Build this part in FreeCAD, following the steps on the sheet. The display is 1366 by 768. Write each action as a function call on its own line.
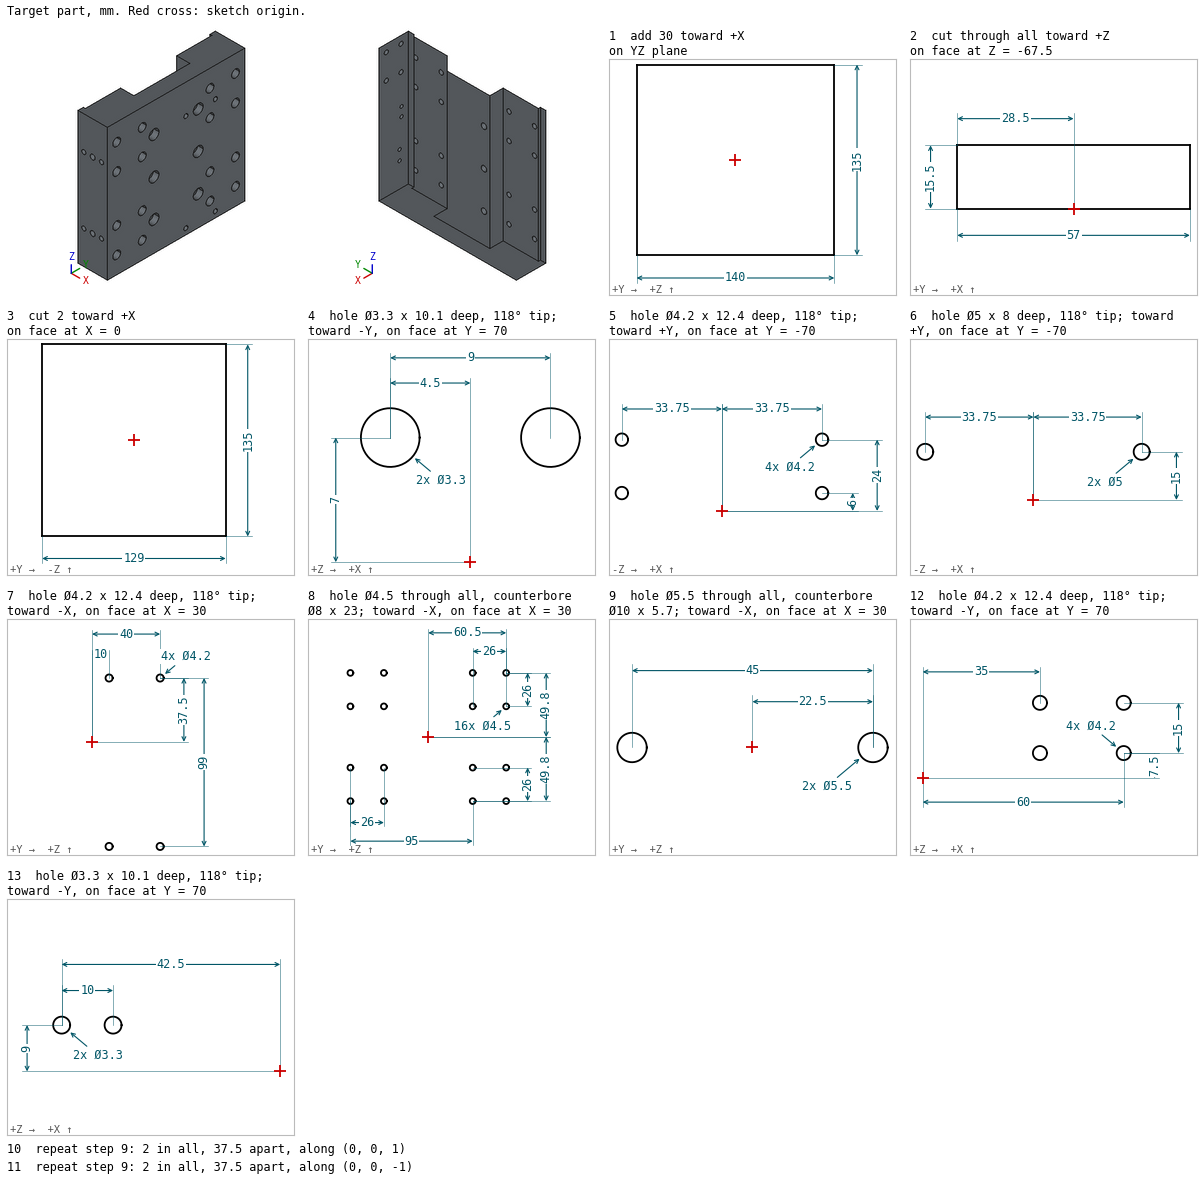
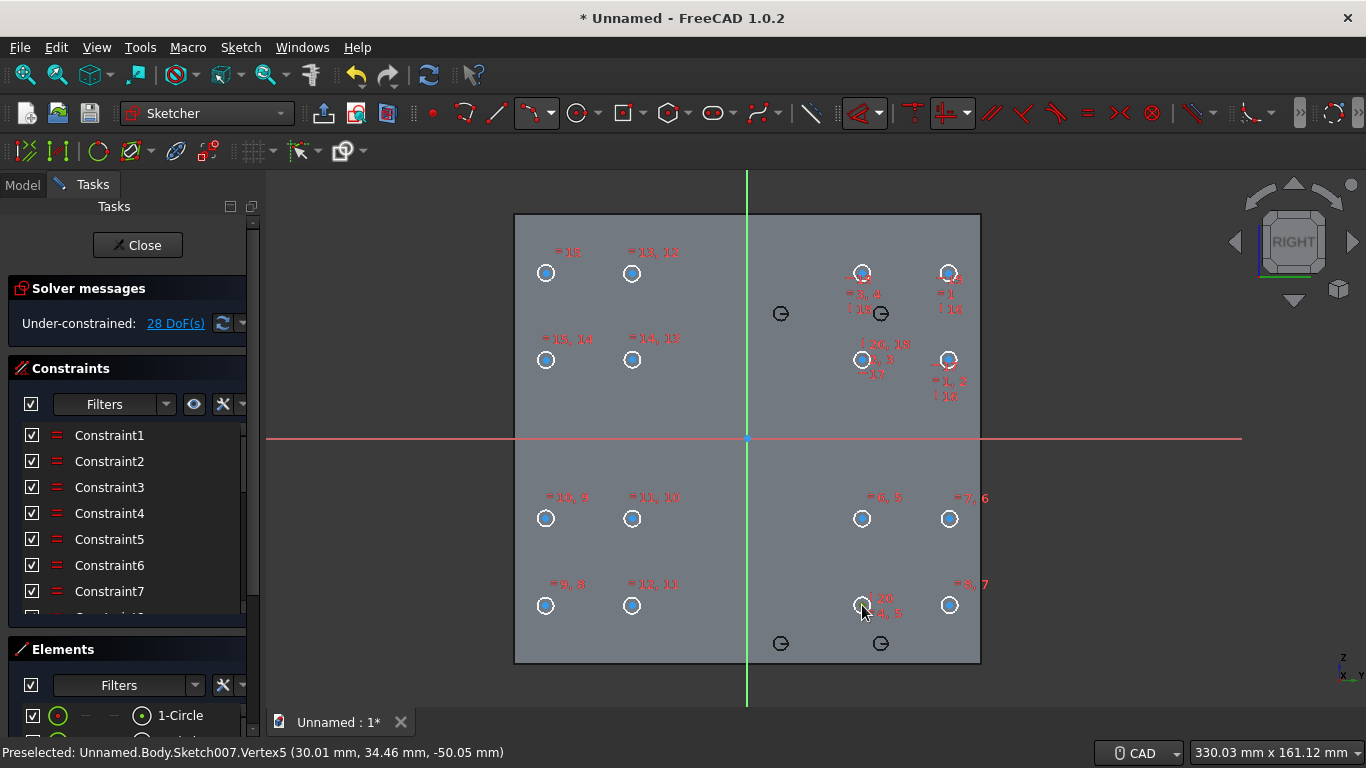
click(862, 519)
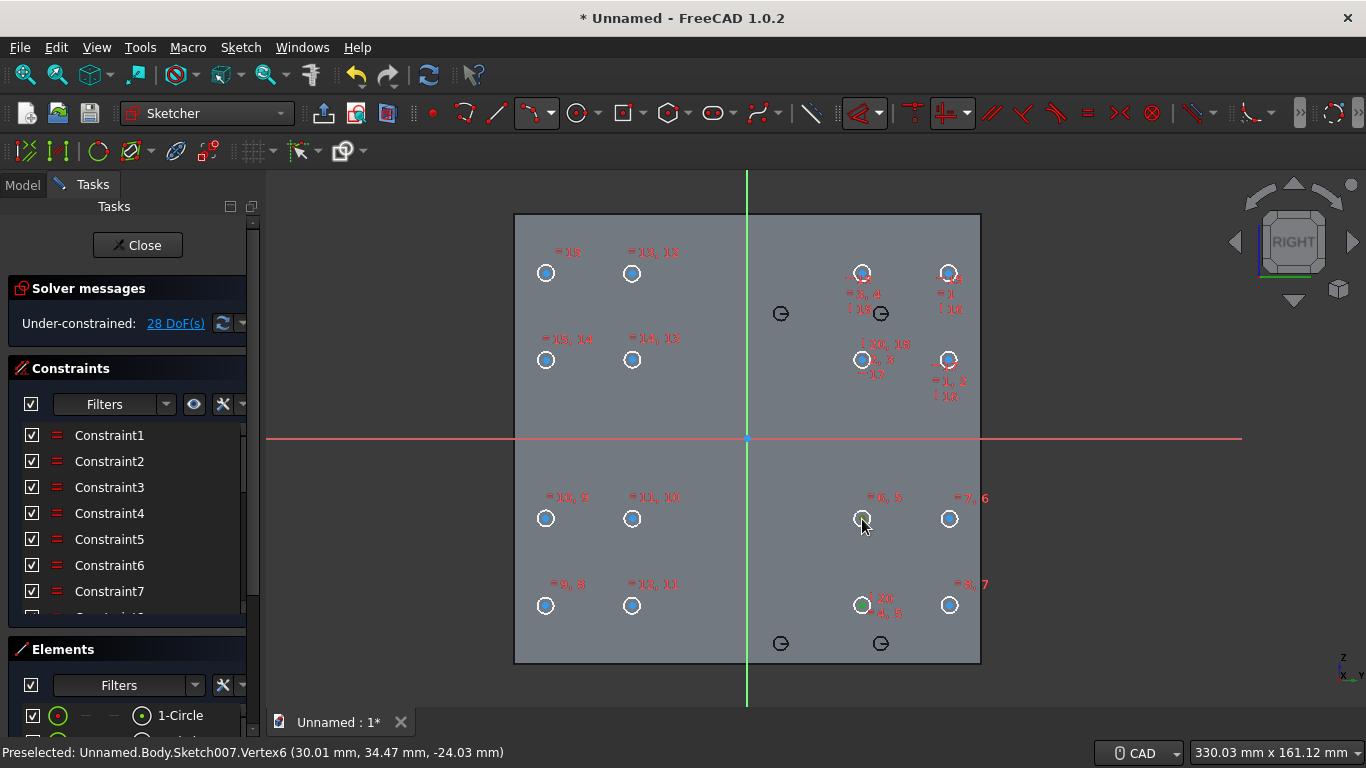
click(970, 114)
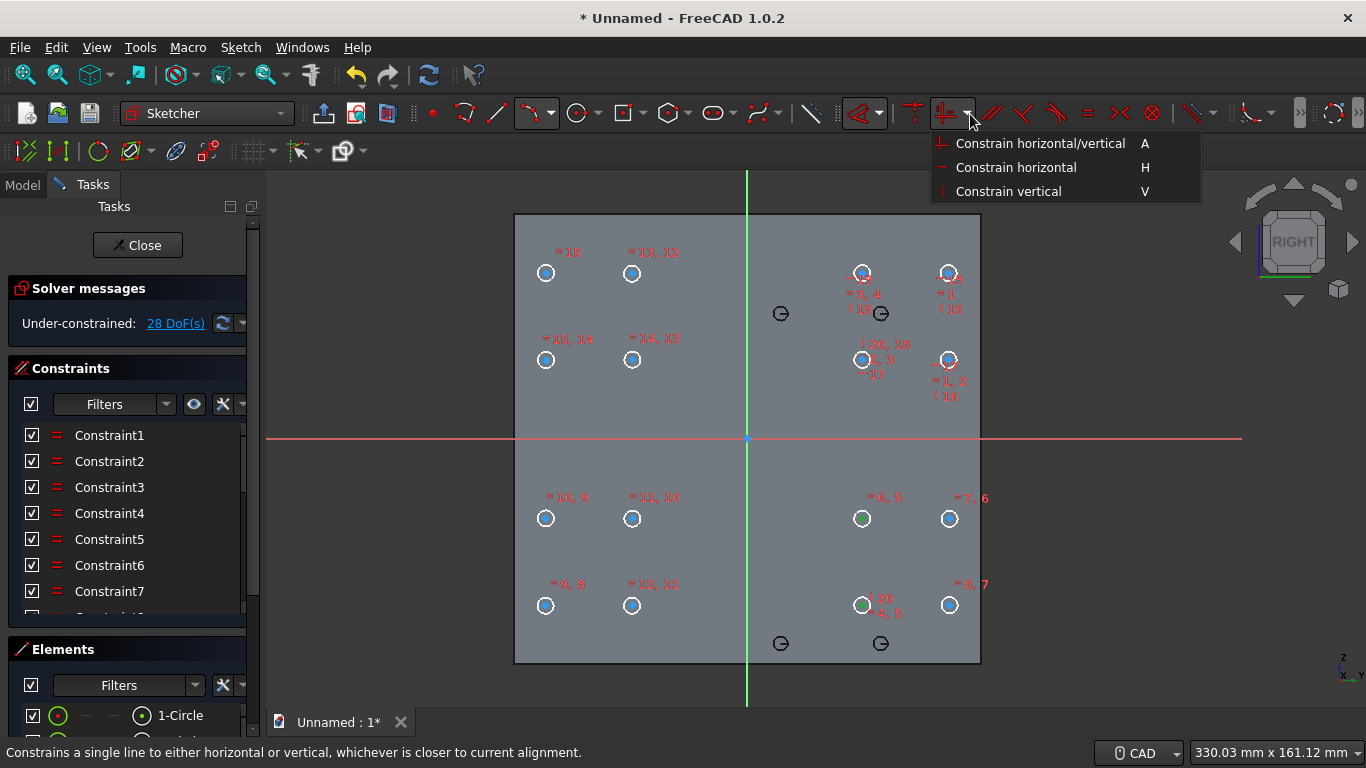
click(1066, 191)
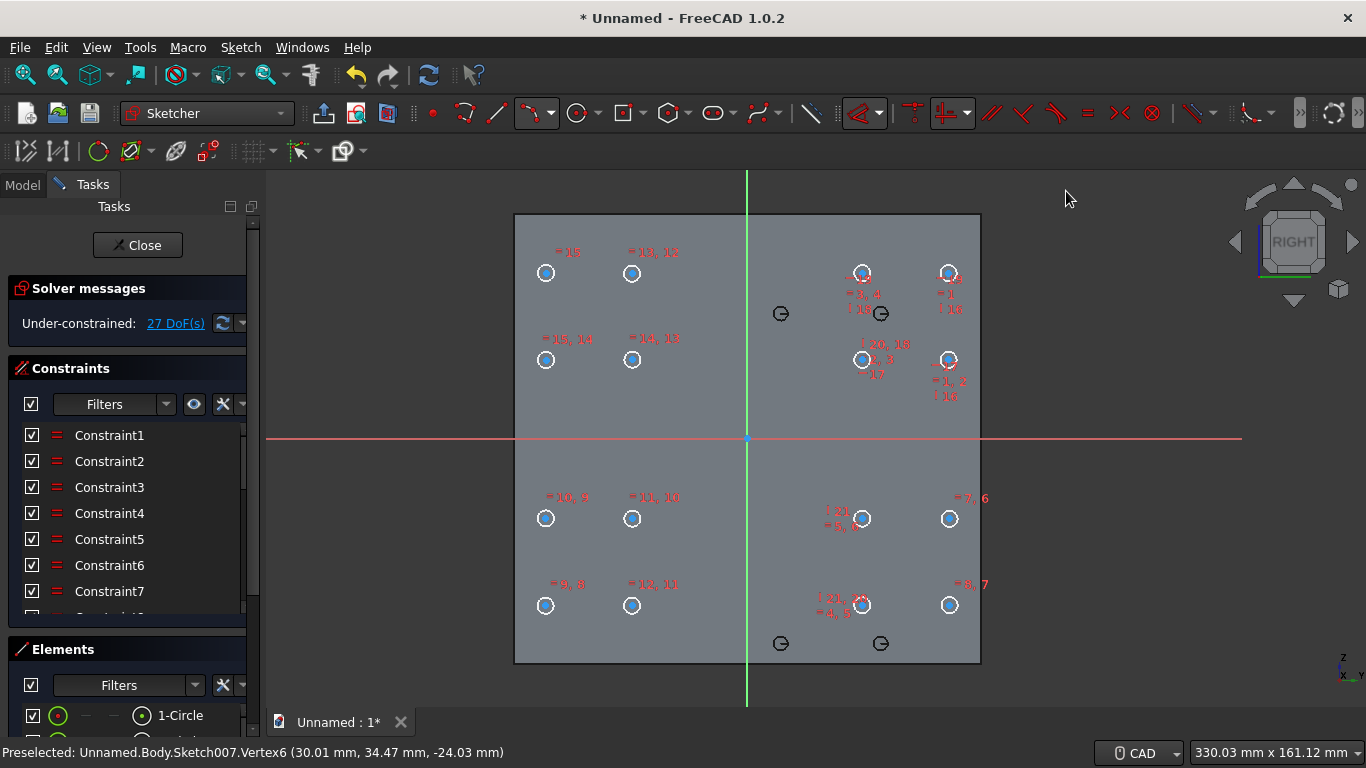
click(949, 360)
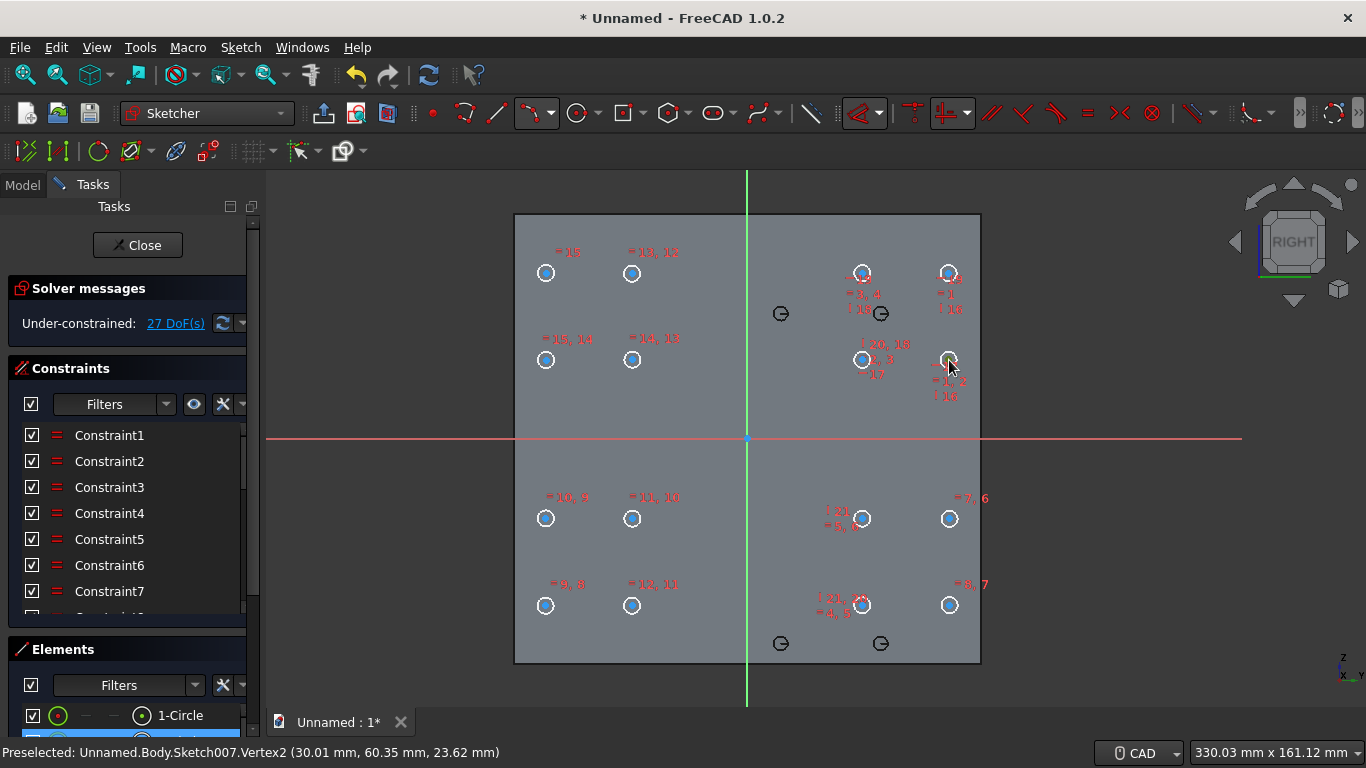
click(950, 519)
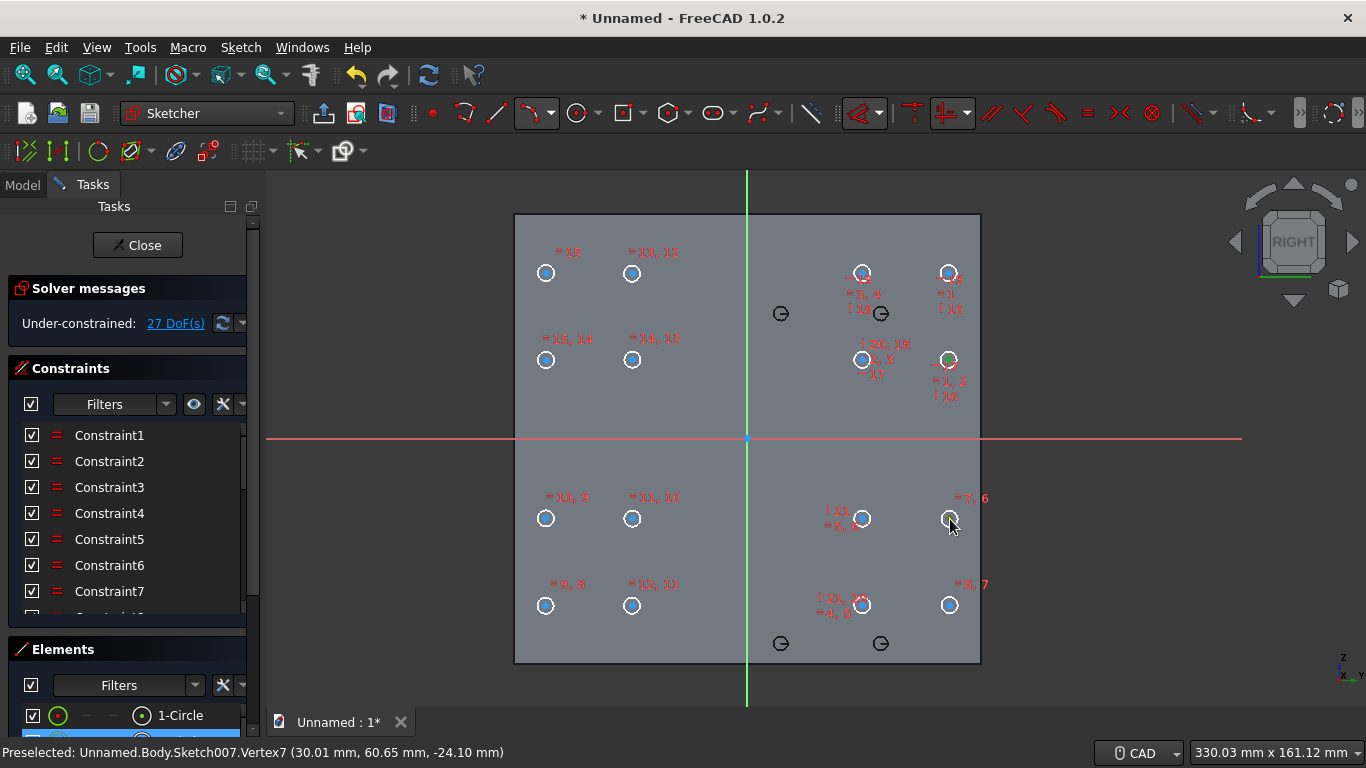
key(v)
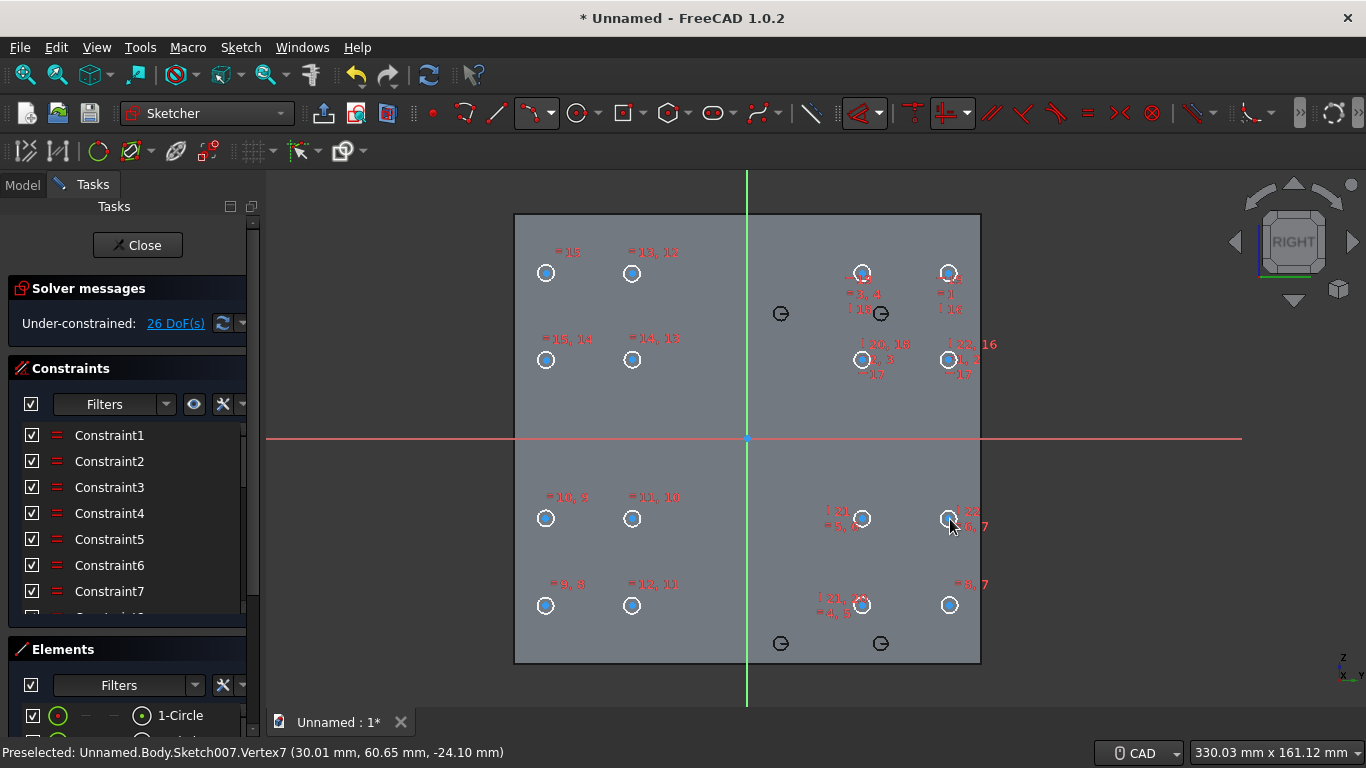
click(862, 519)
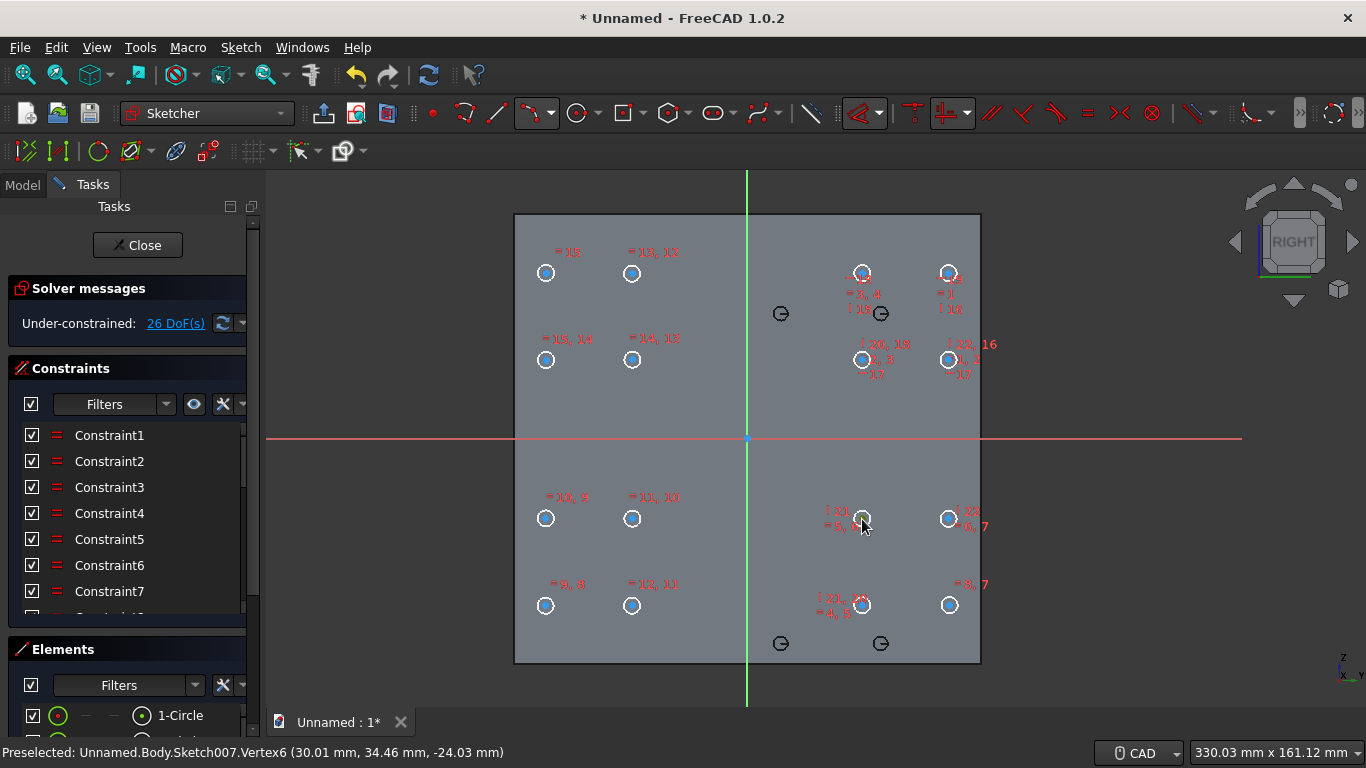
click(949, 519)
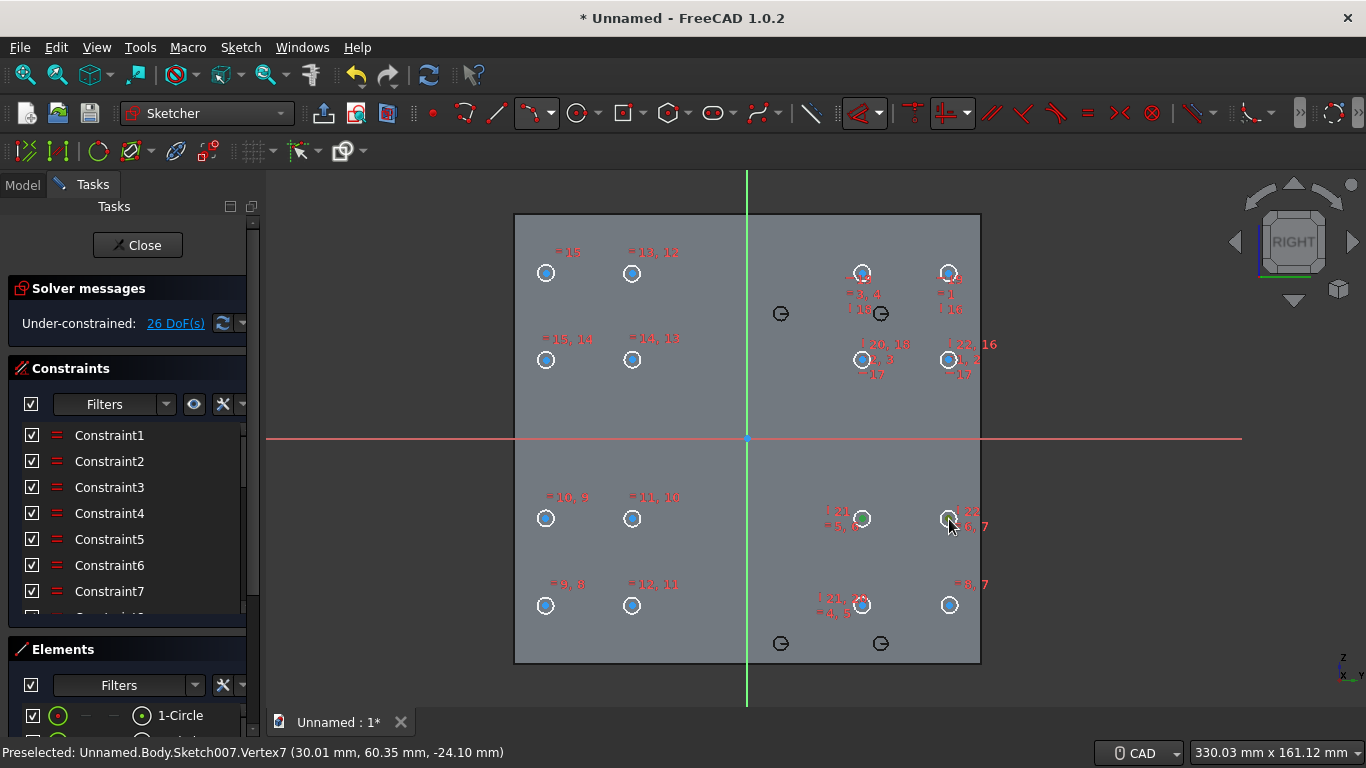
click(970, 114)